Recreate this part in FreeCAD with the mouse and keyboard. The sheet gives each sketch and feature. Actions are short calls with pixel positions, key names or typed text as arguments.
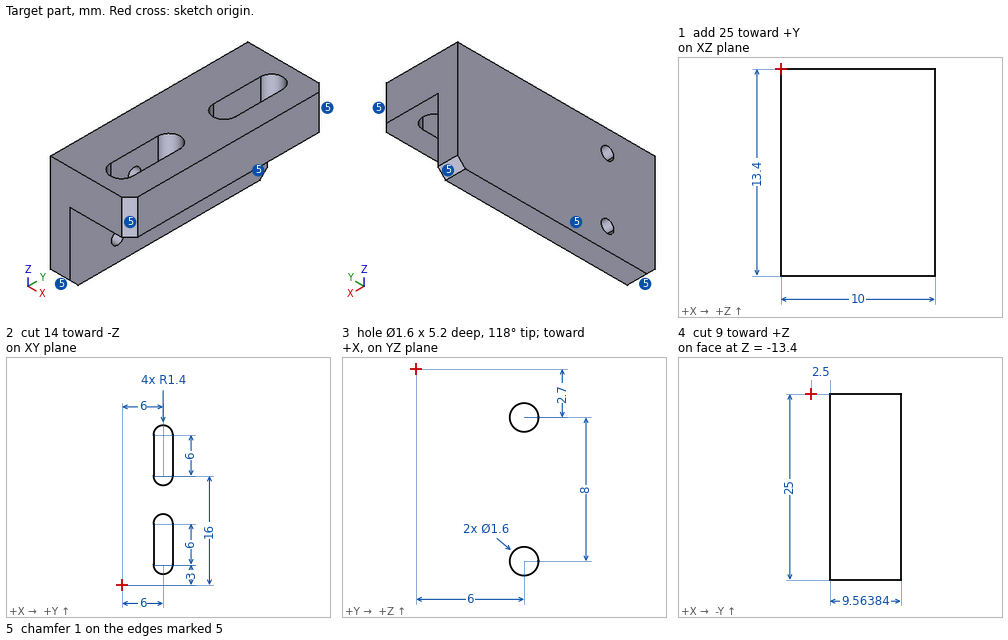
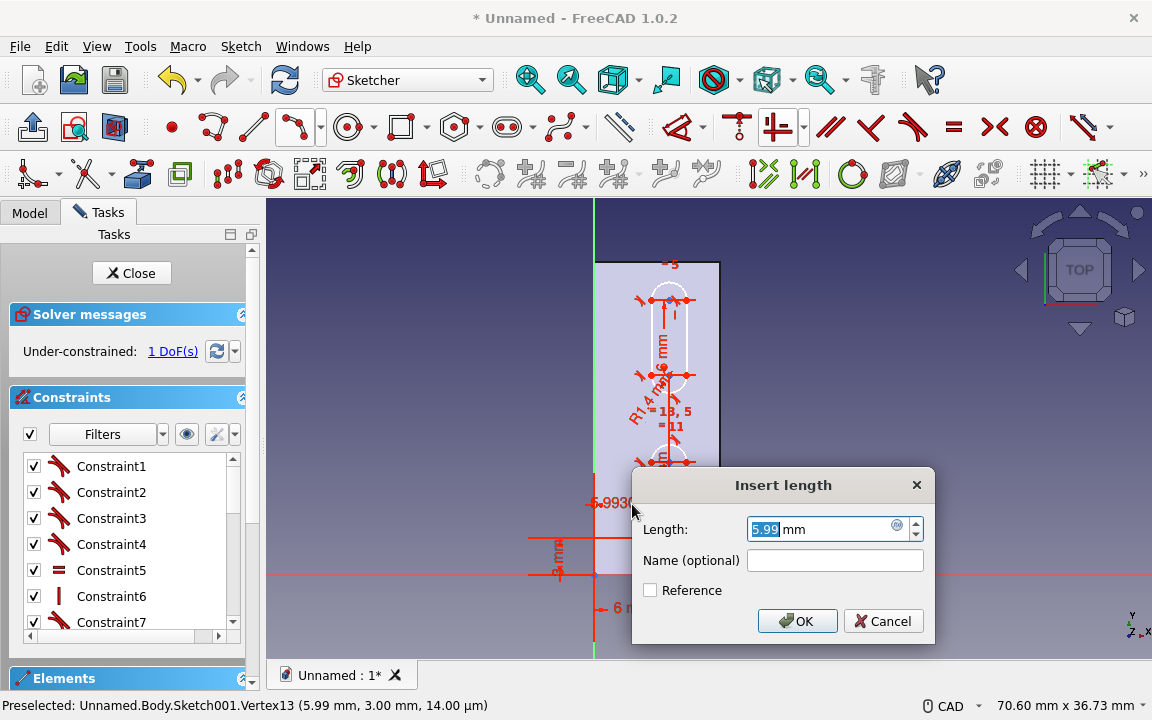
text(6)
key(Return)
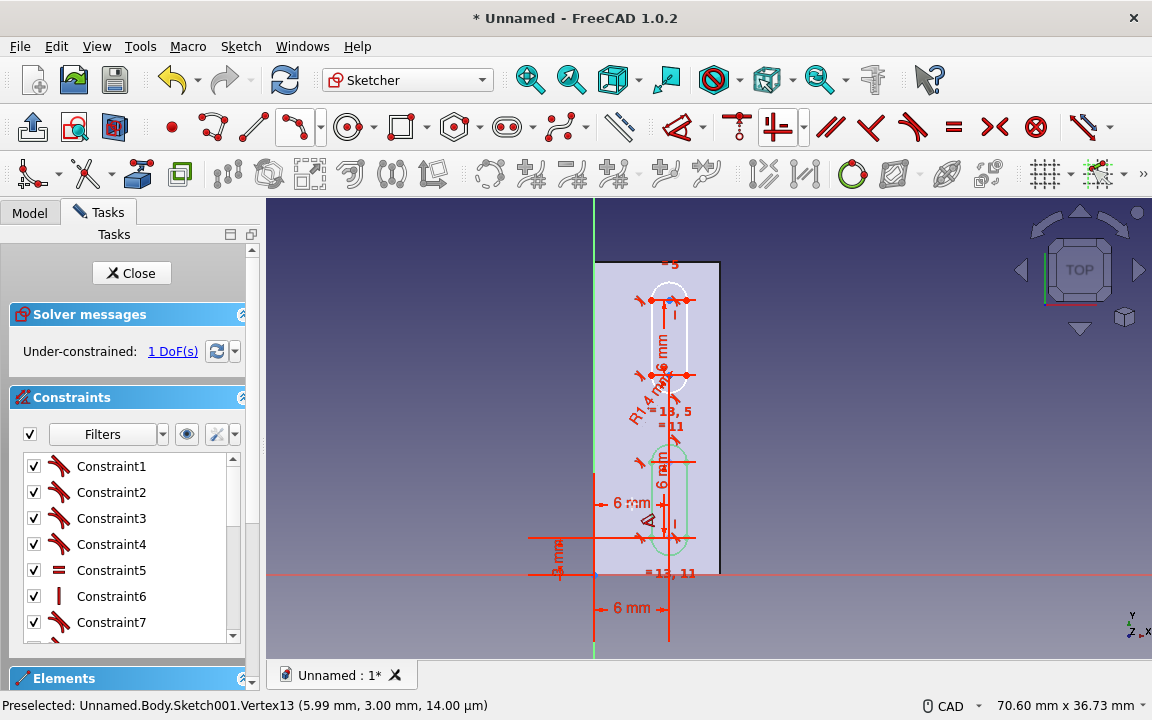
click(652, 375)
click(560, 475)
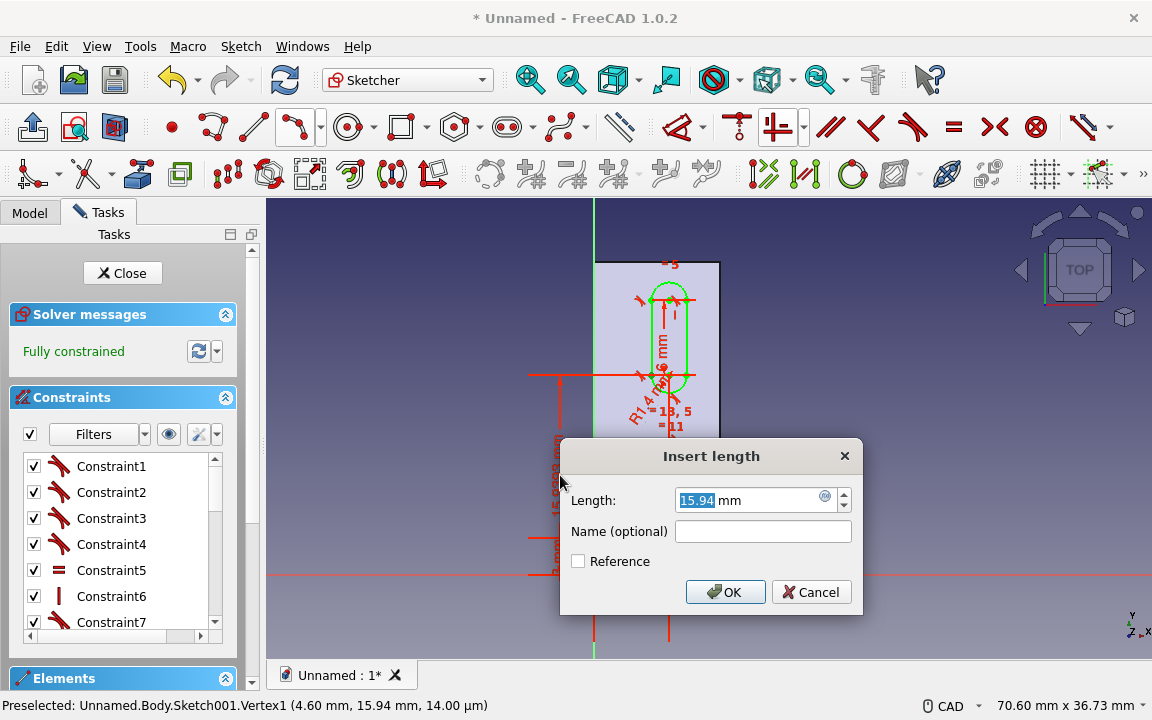
text(16)
key(Return)
key(Escape)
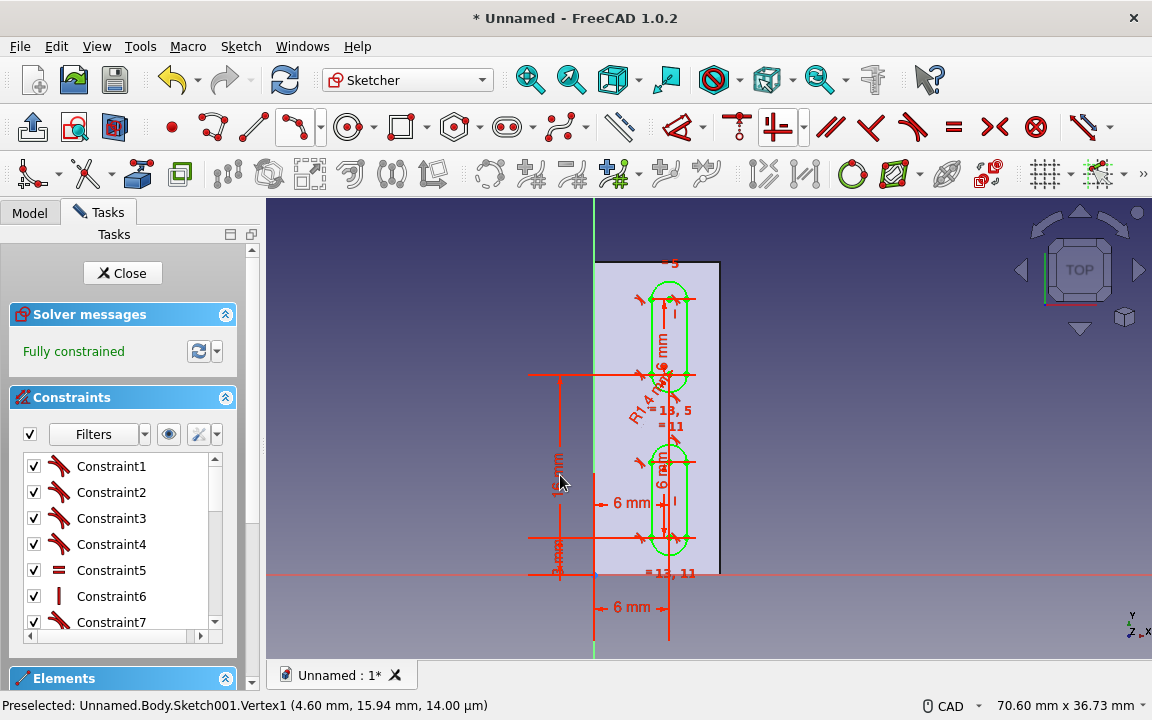
click(123, 273)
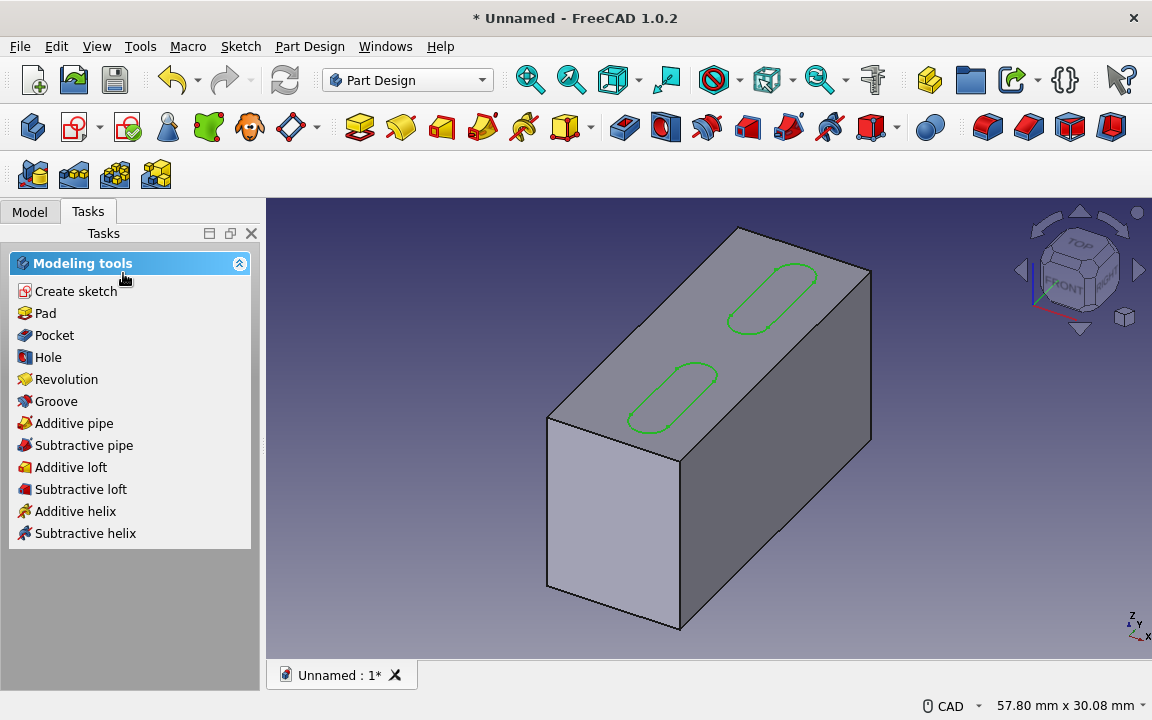
click(625, 128)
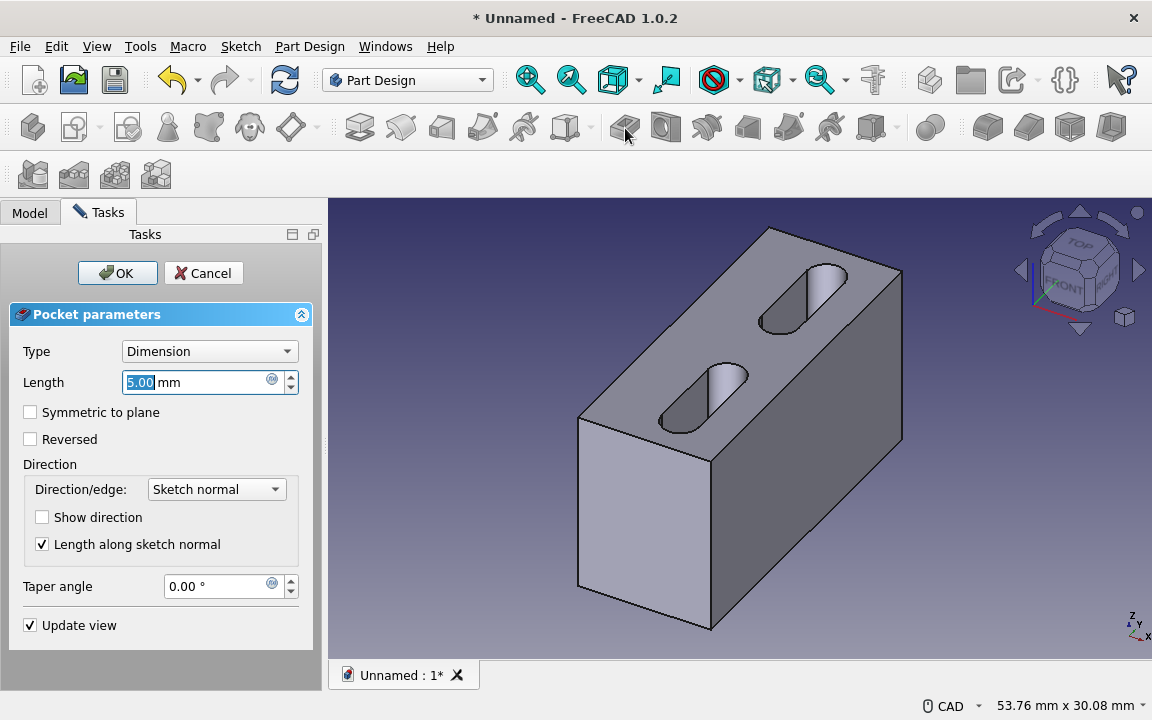
text(14)
key(Tab)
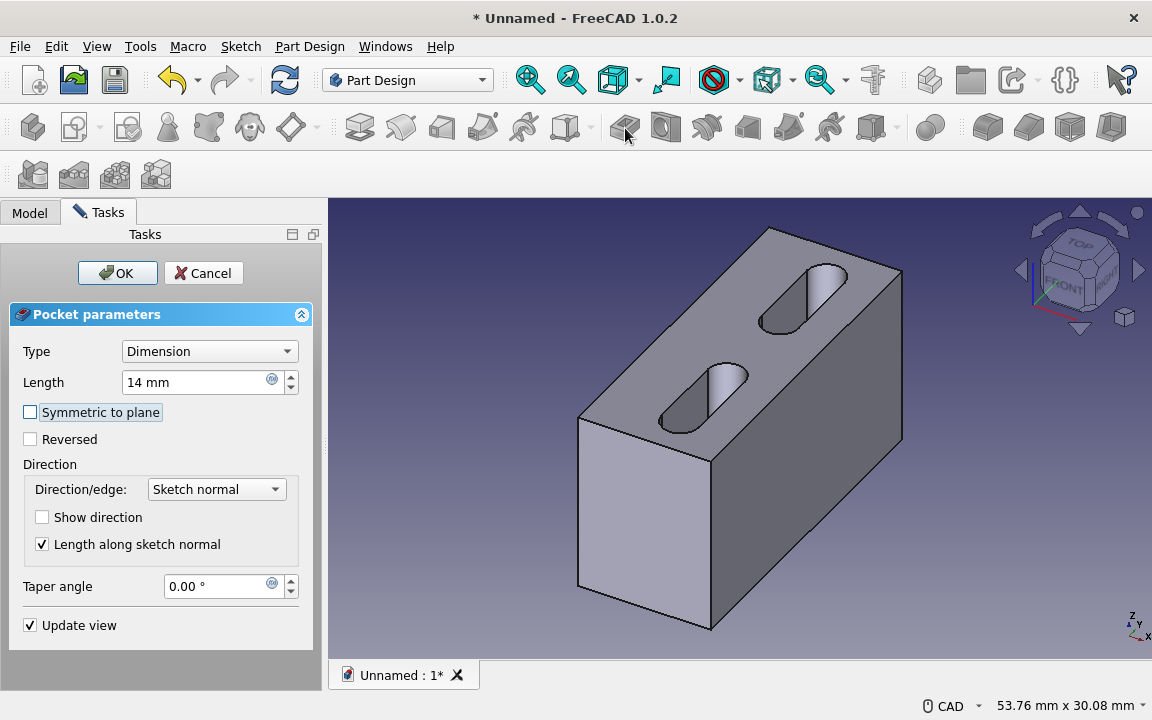
click(118, 273)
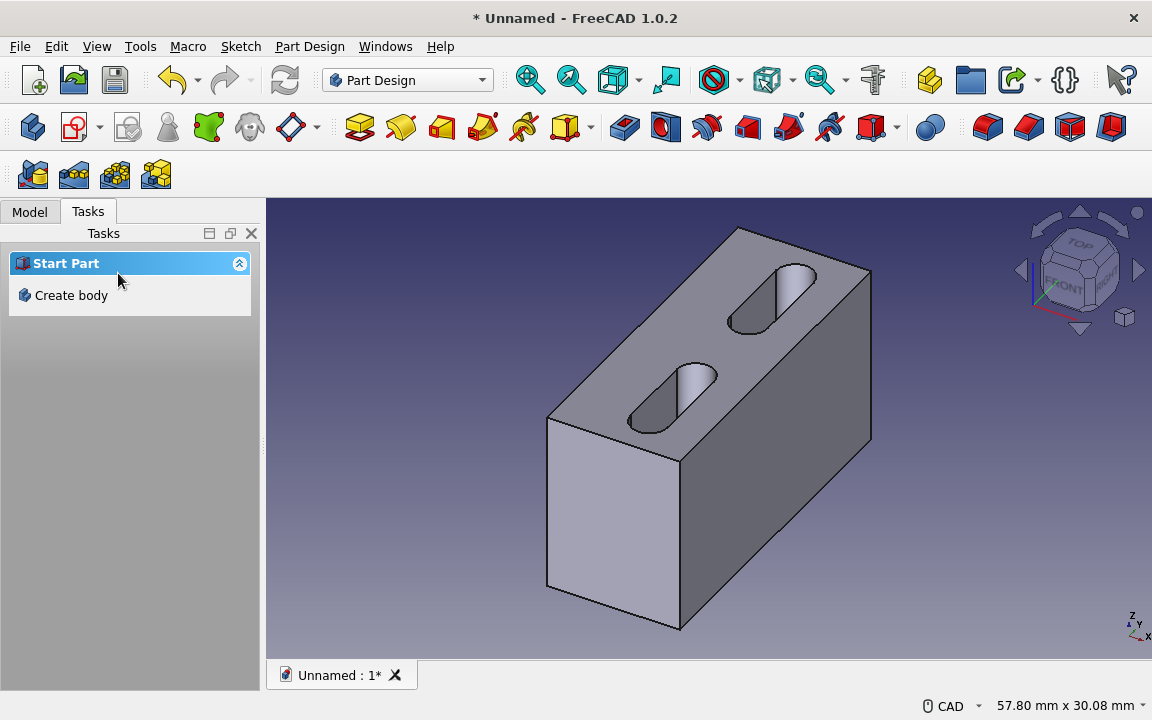
click(74, 128)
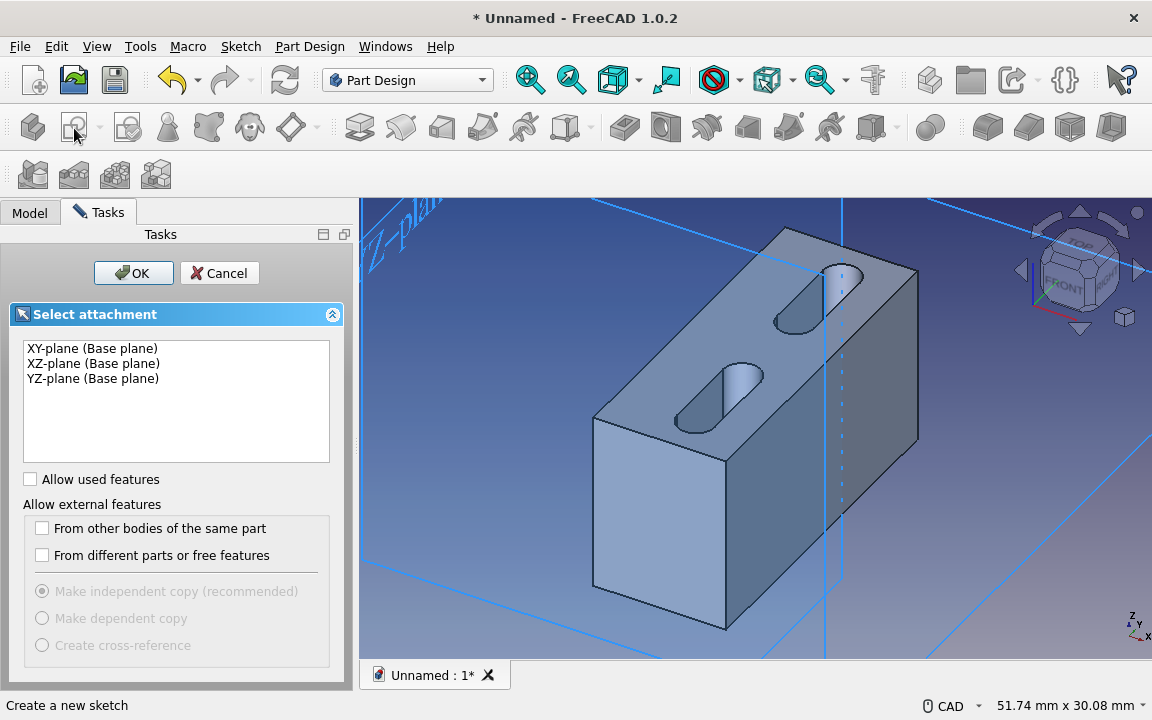
click(84, 378)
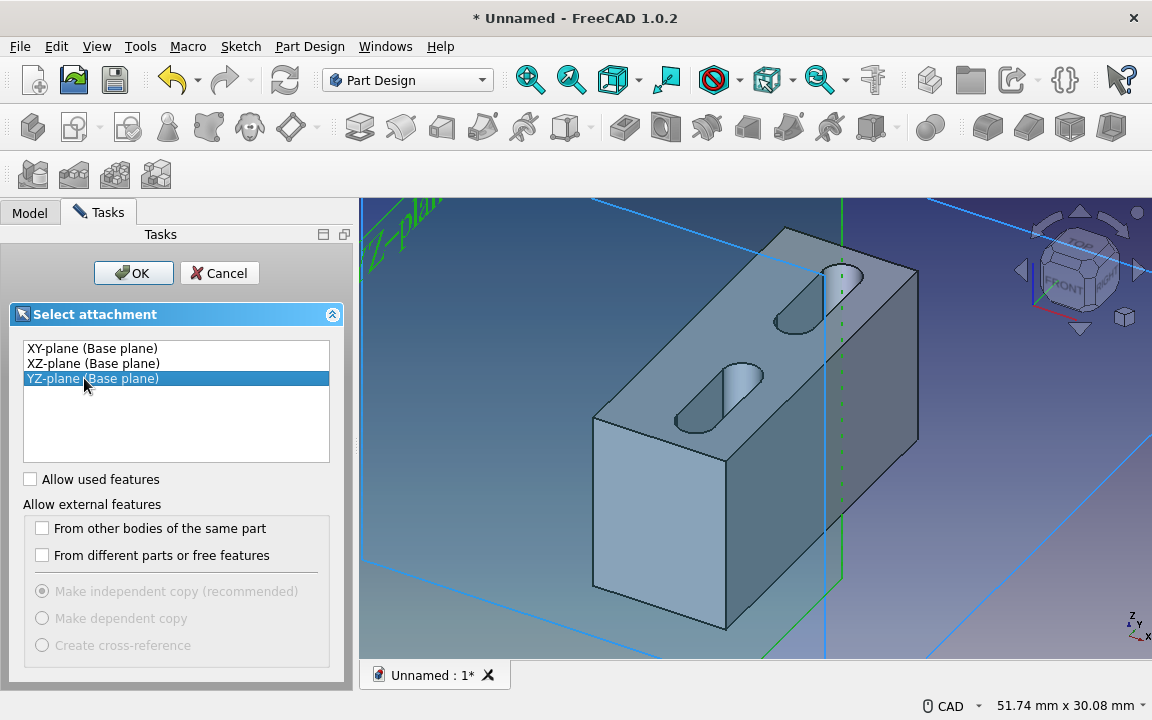
click(134, 273)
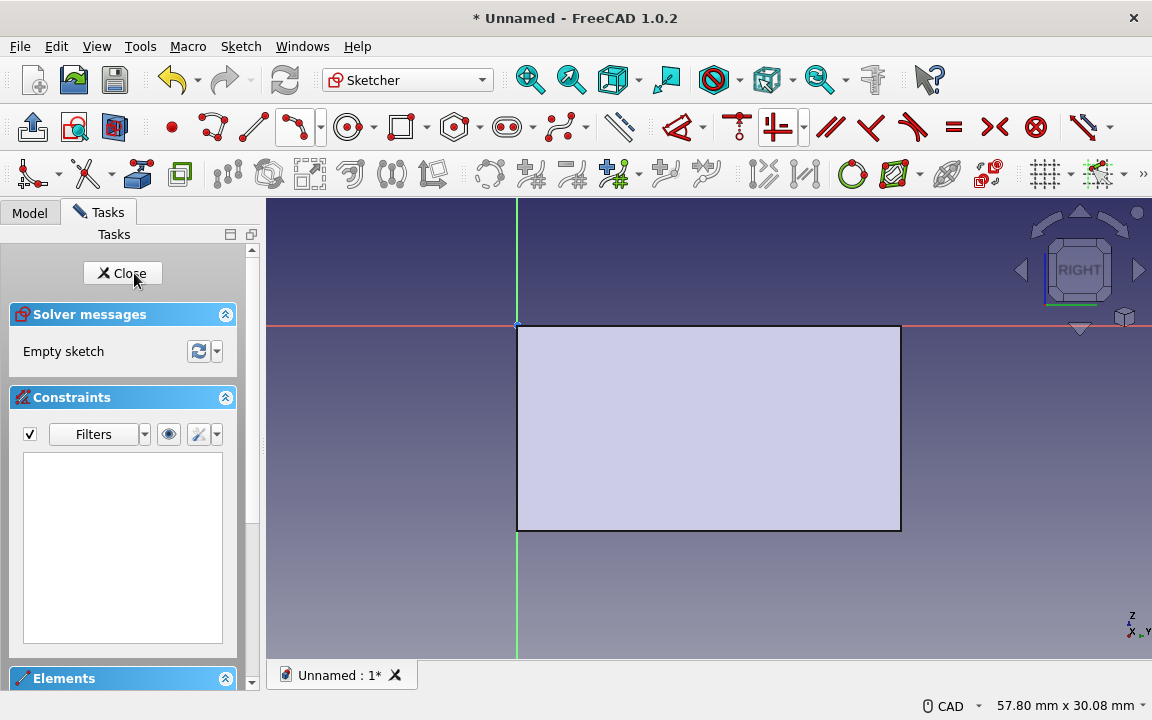
click(115, 128)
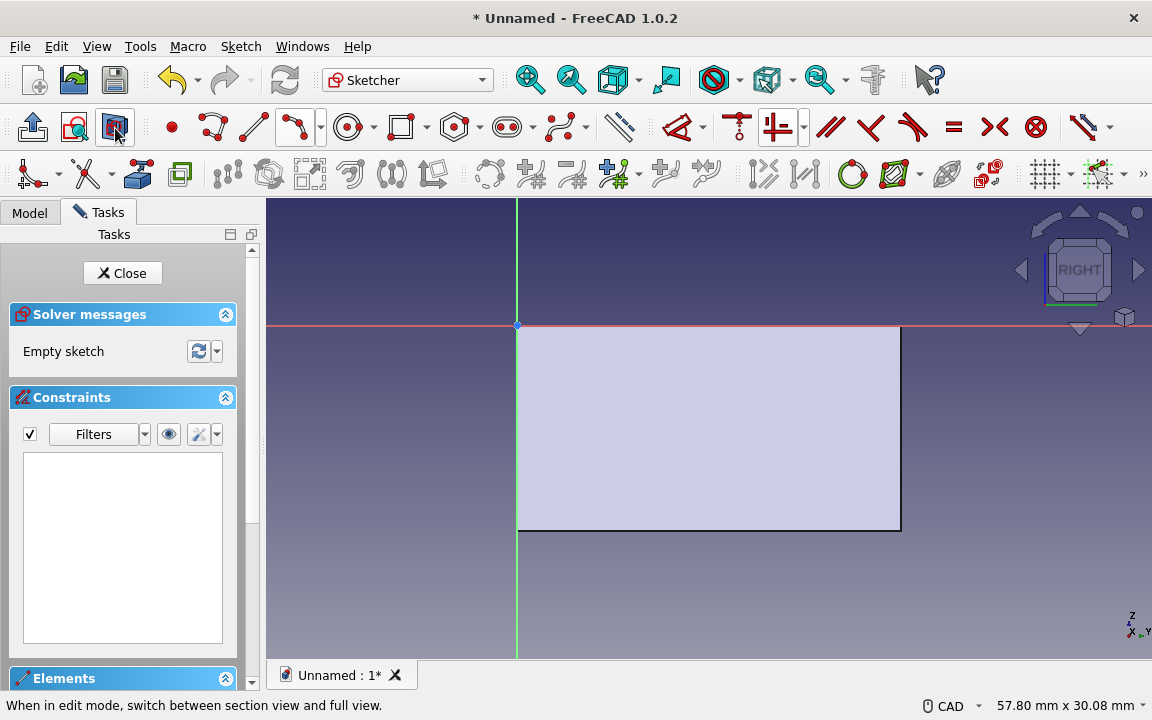
scroll(425, 384, up, 2)